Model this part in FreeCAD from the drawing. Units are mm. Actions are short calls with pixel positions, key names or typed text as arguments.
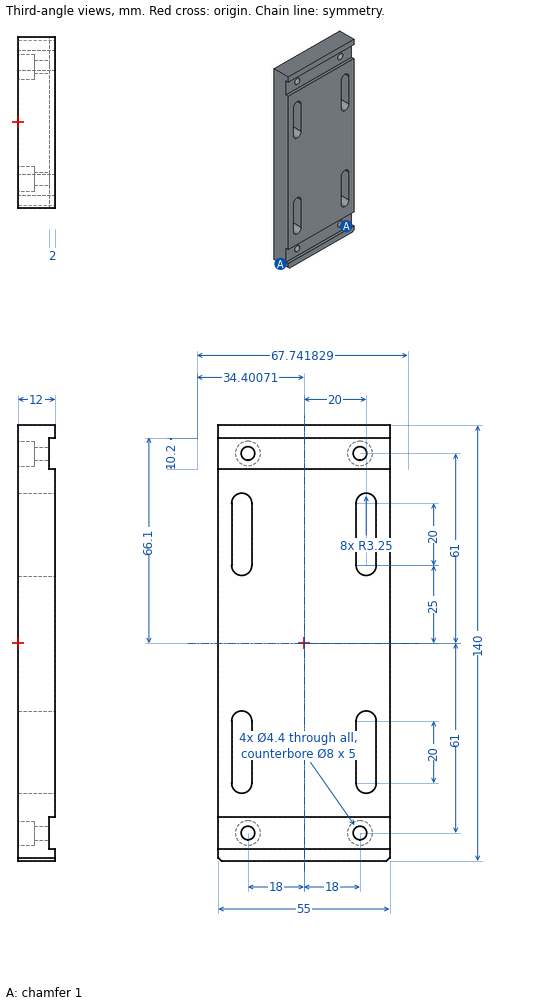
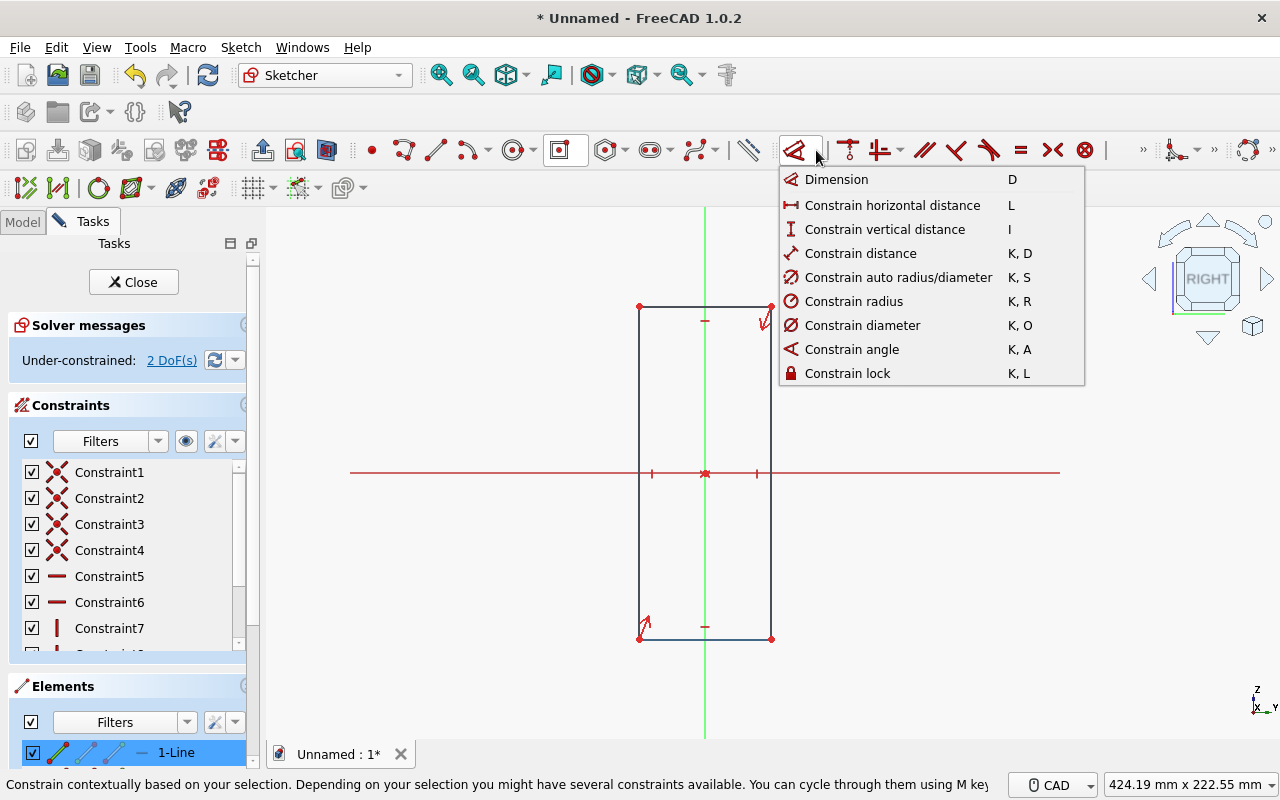
click(932, 205)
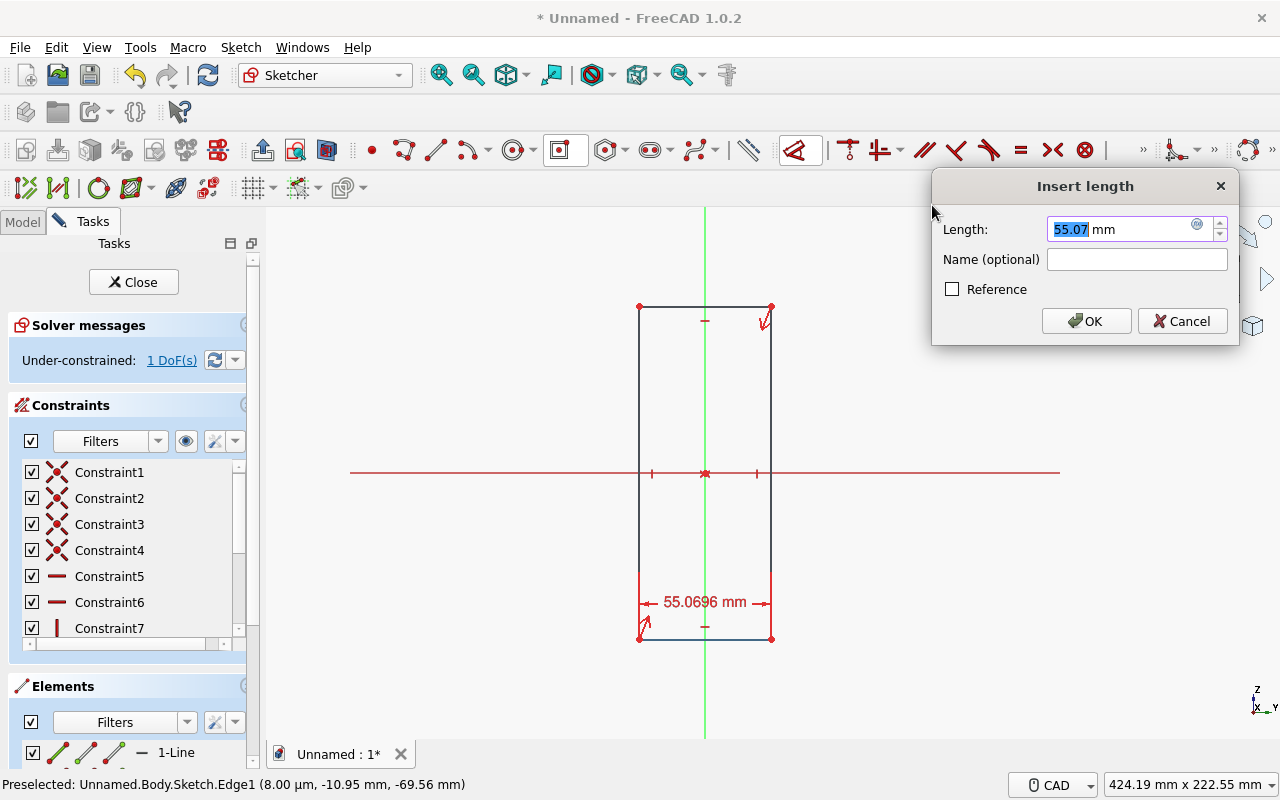
text(55)
key(Return)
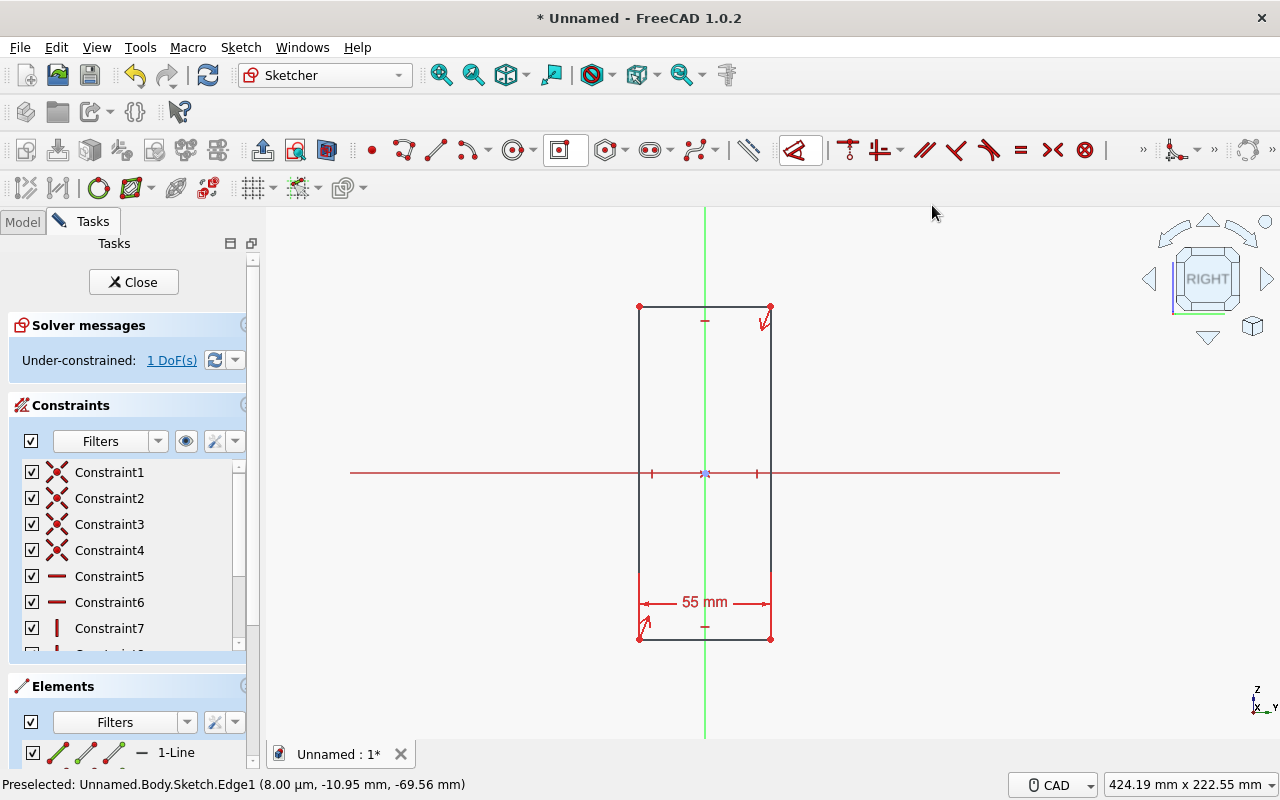
click(771, 540)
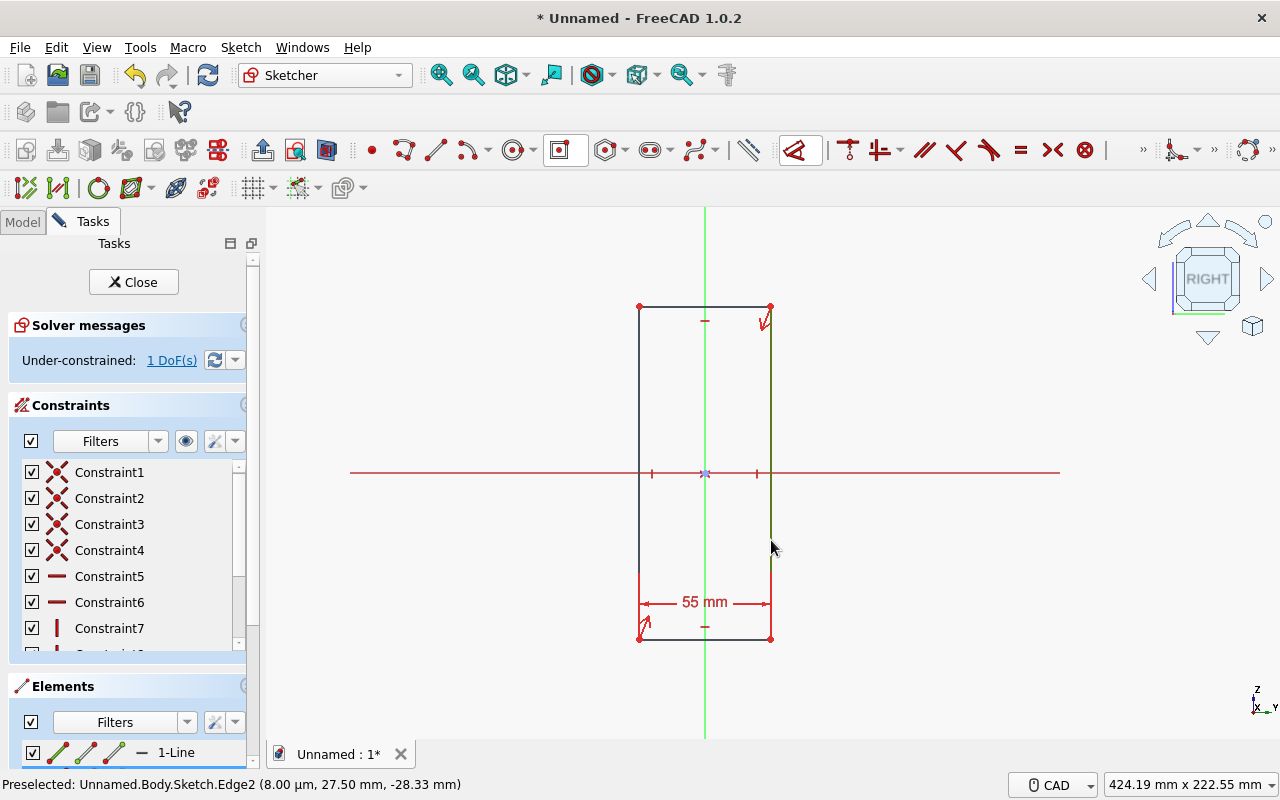
click(816, 150)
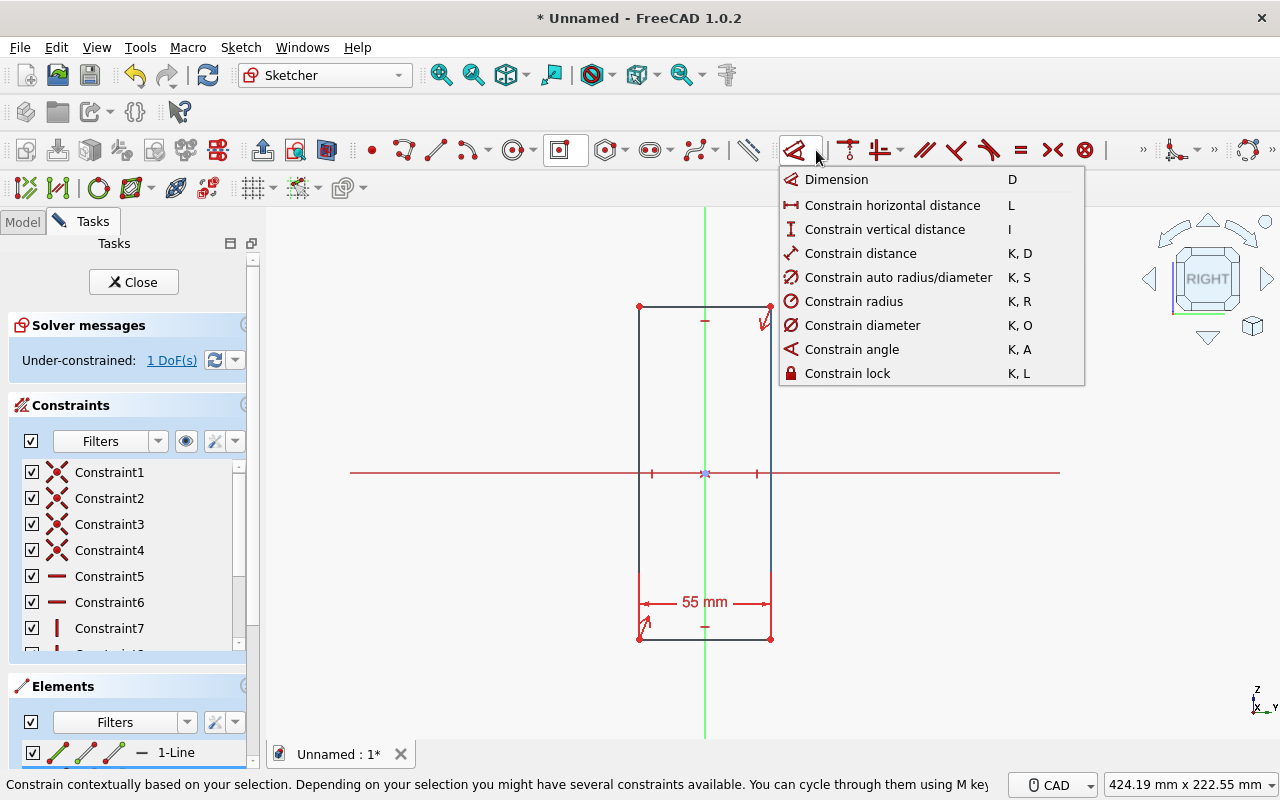
click(932, 229)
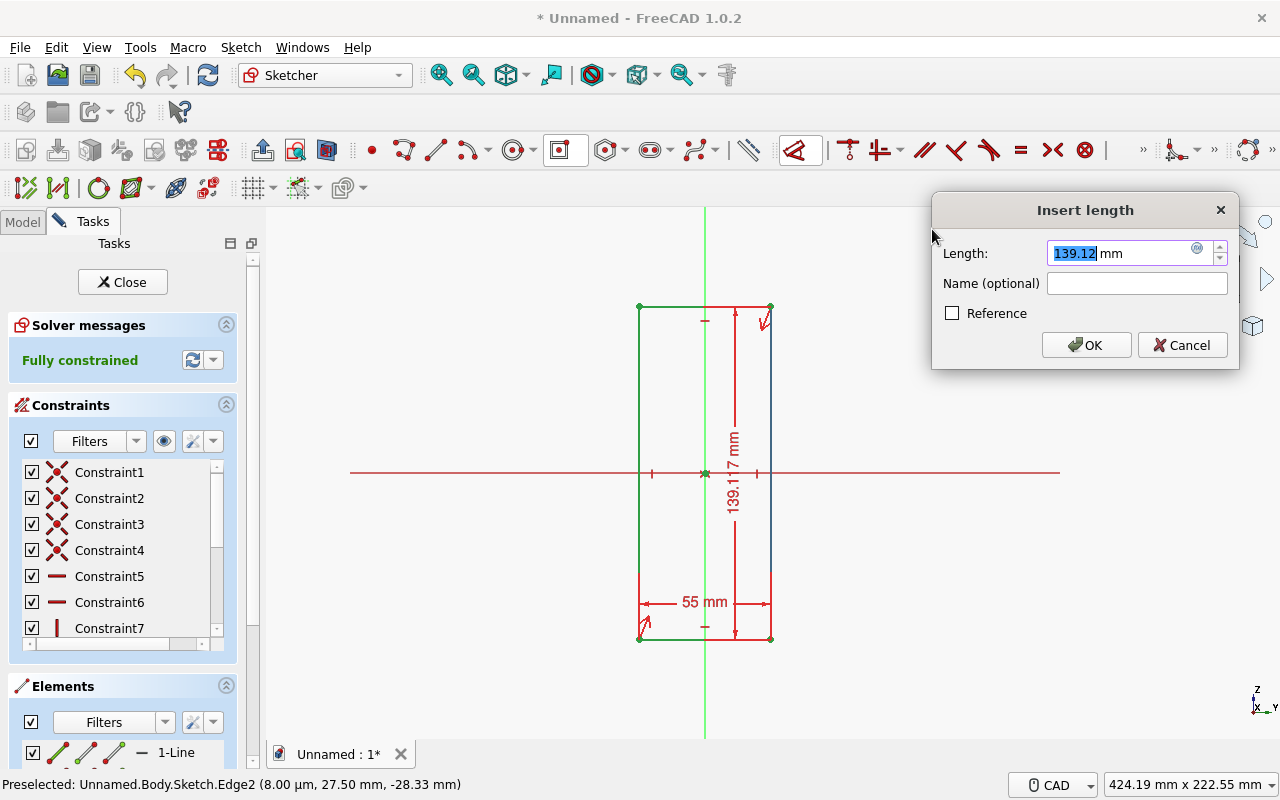
text(140)
key(Return)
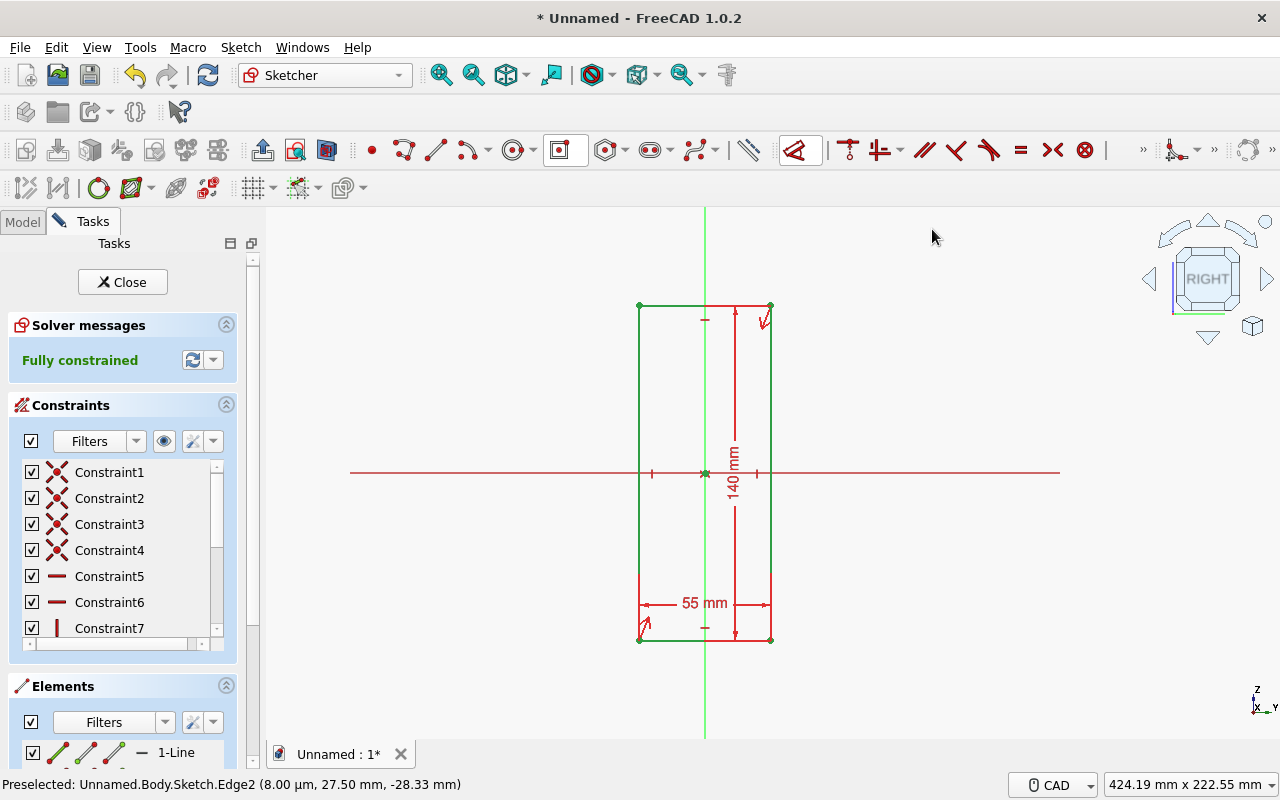
click(123, 282)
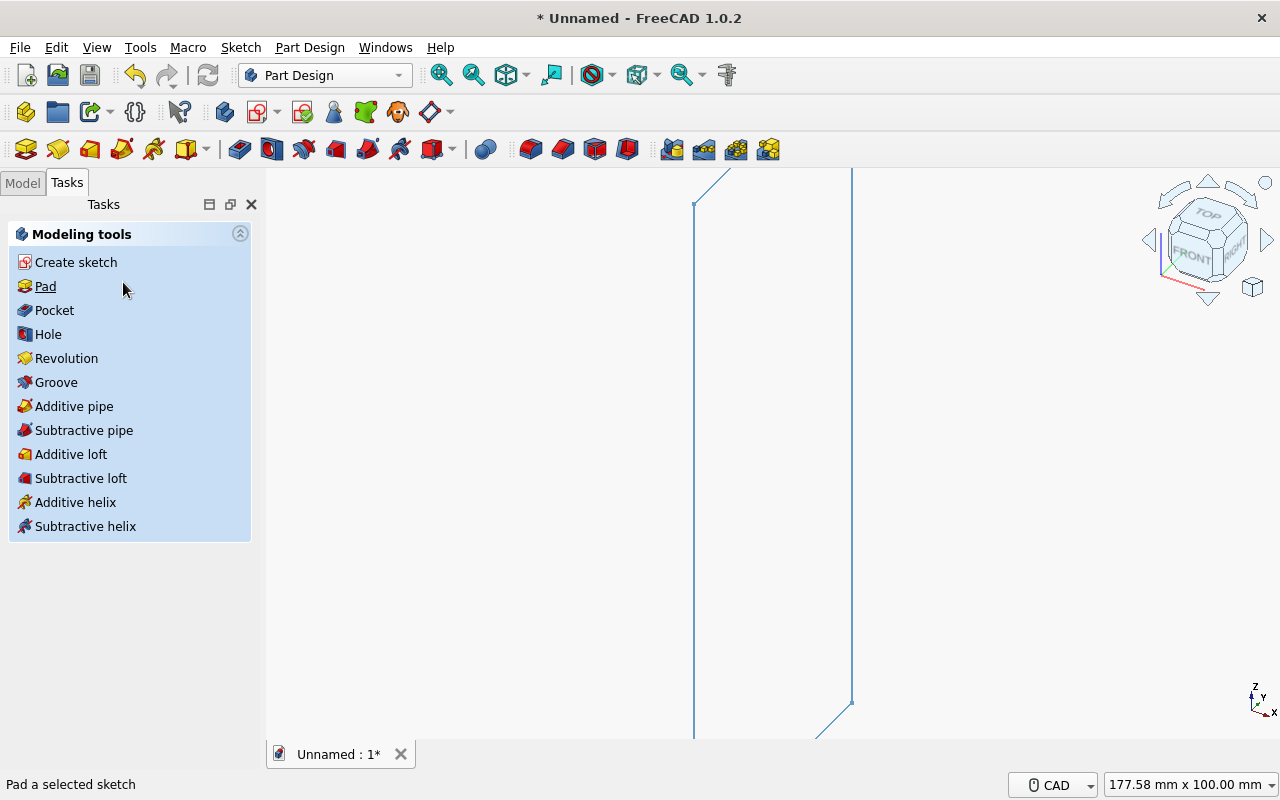
click(26, 150)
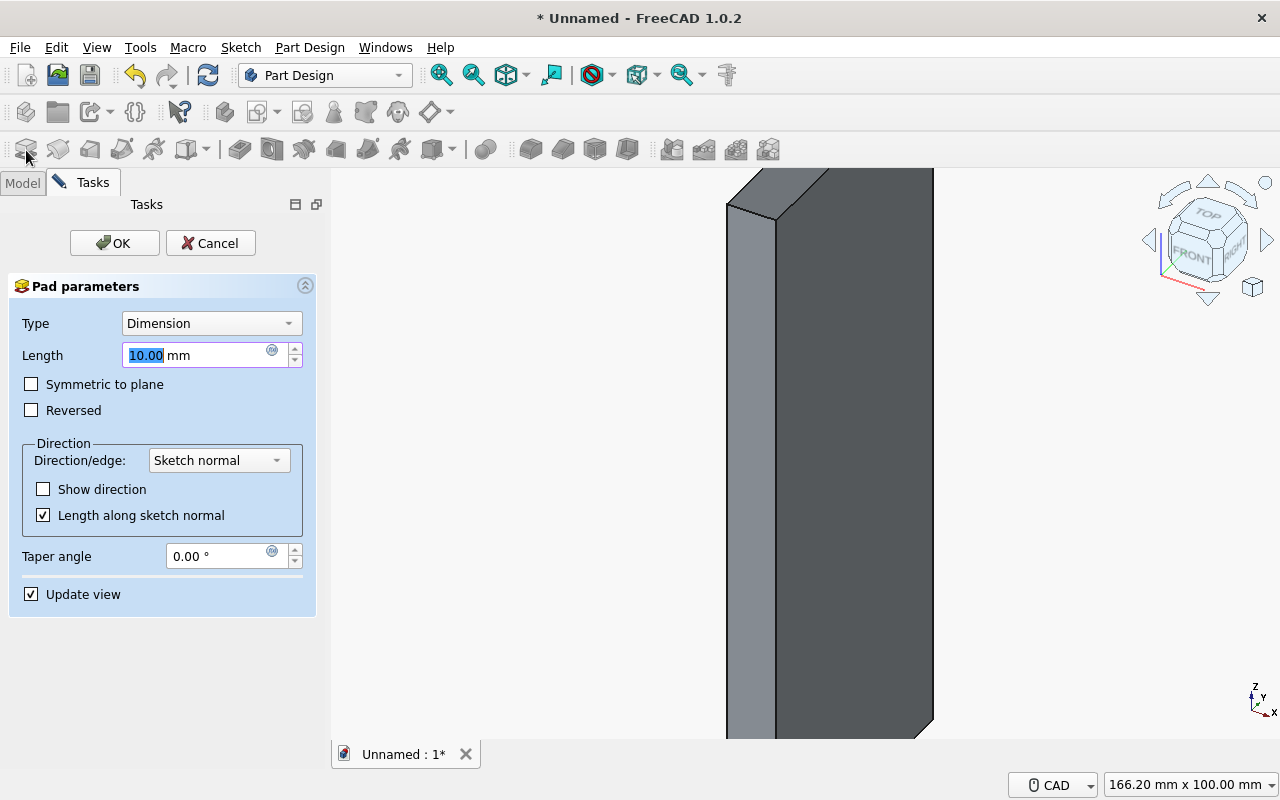
text(12)
key(Tab)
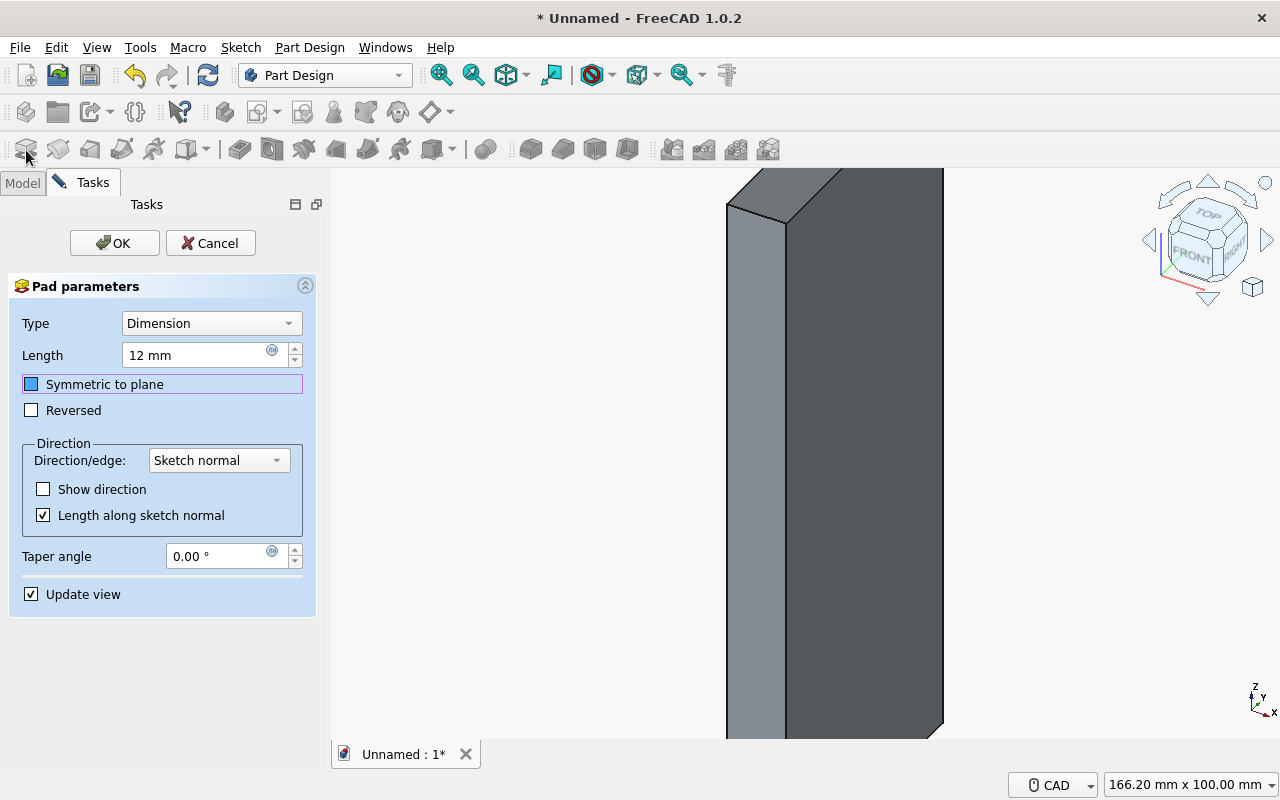
click(115, 243)